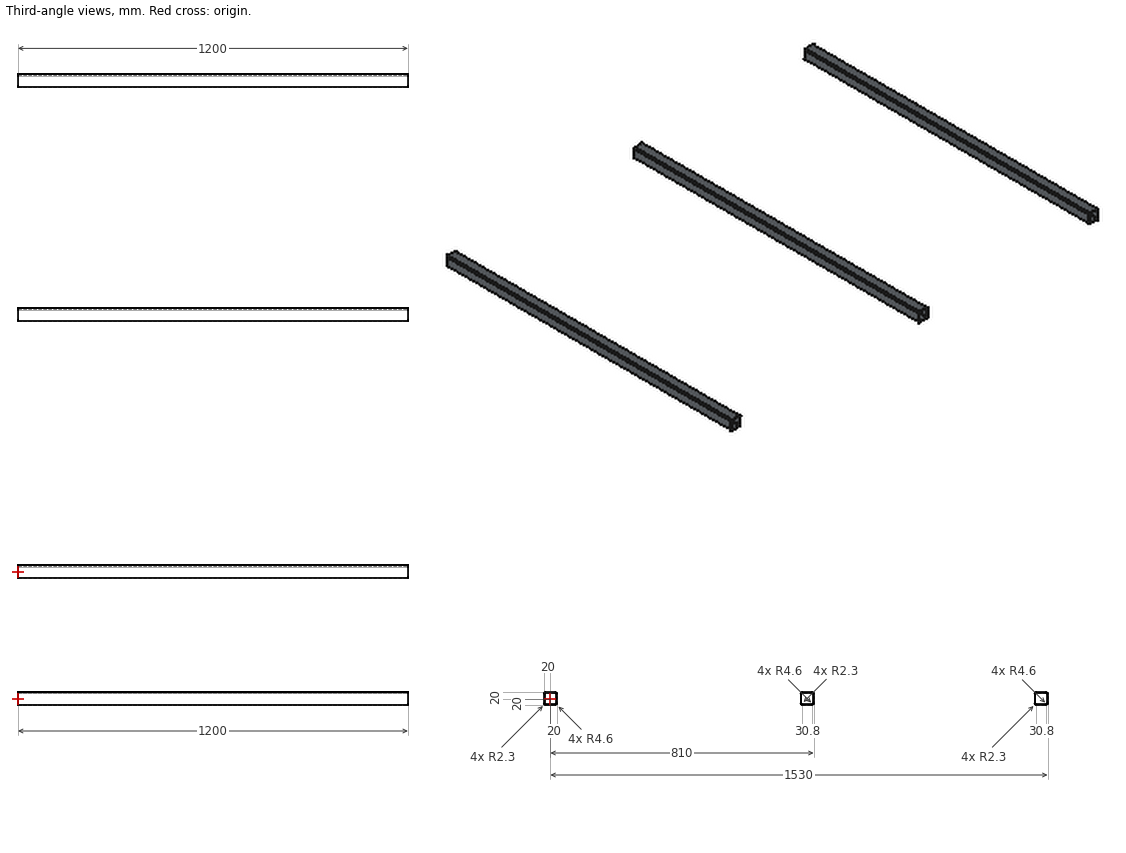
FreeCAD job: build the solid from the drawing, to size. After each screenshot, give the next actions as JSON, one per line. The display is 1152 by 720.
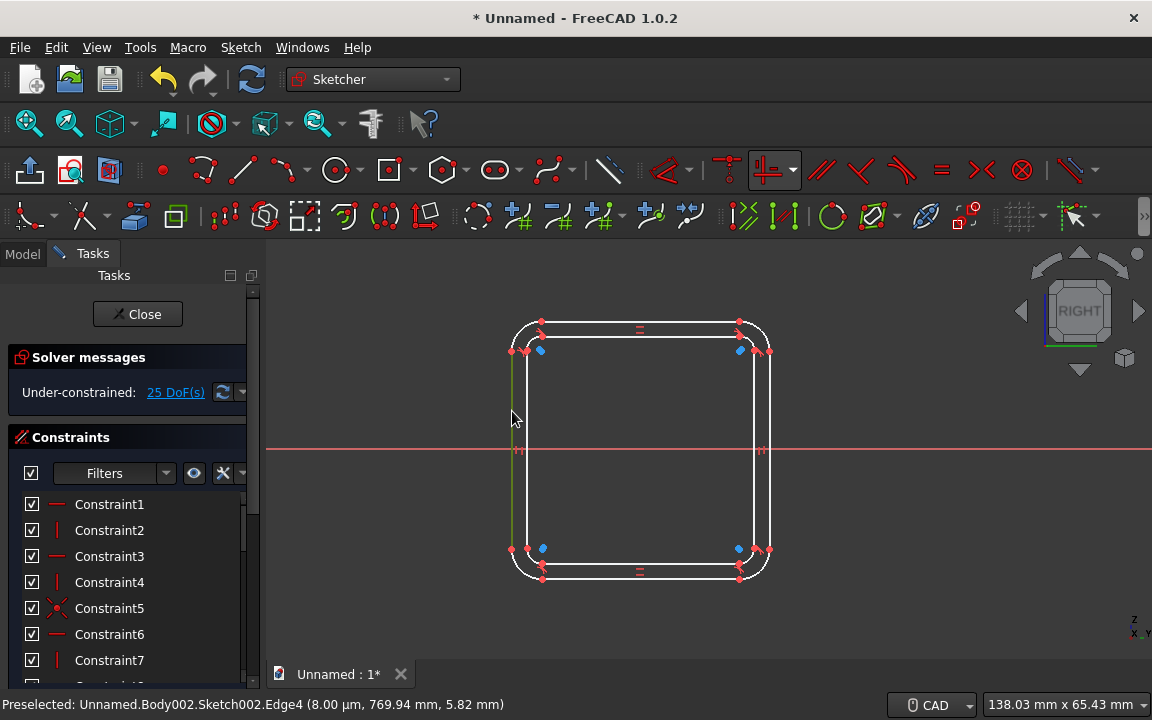
{"action": "left_click", "coordinate": [515, 563]}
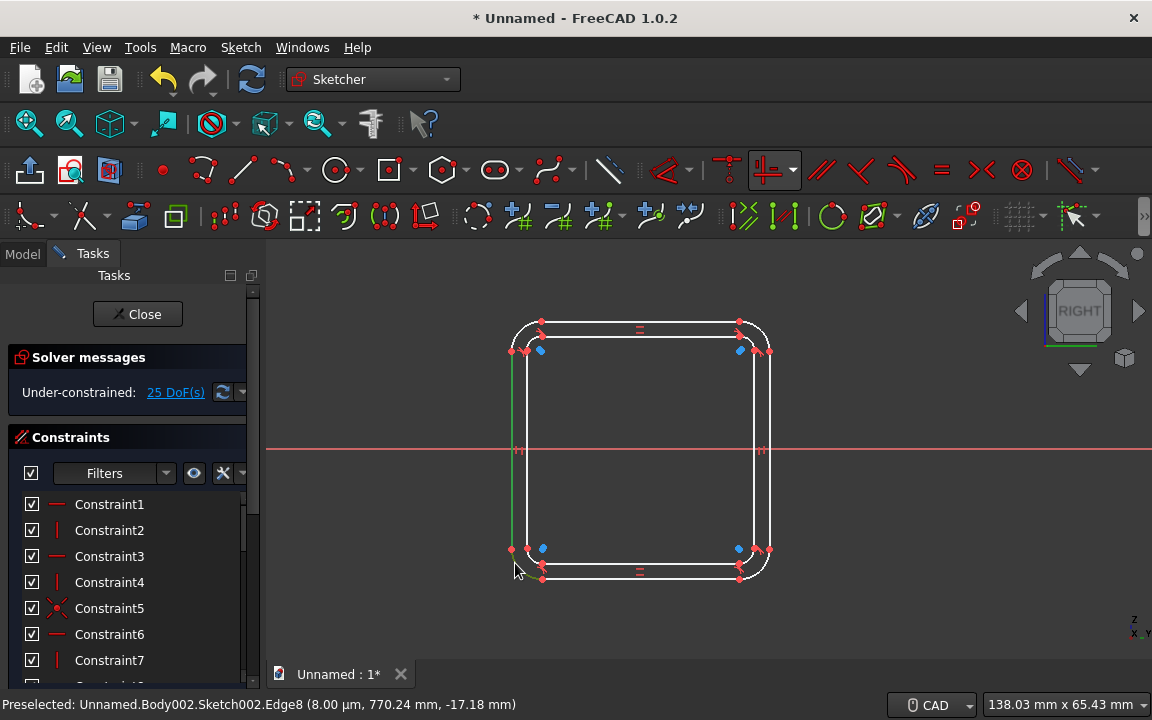
{"action": "key", "text": "t"}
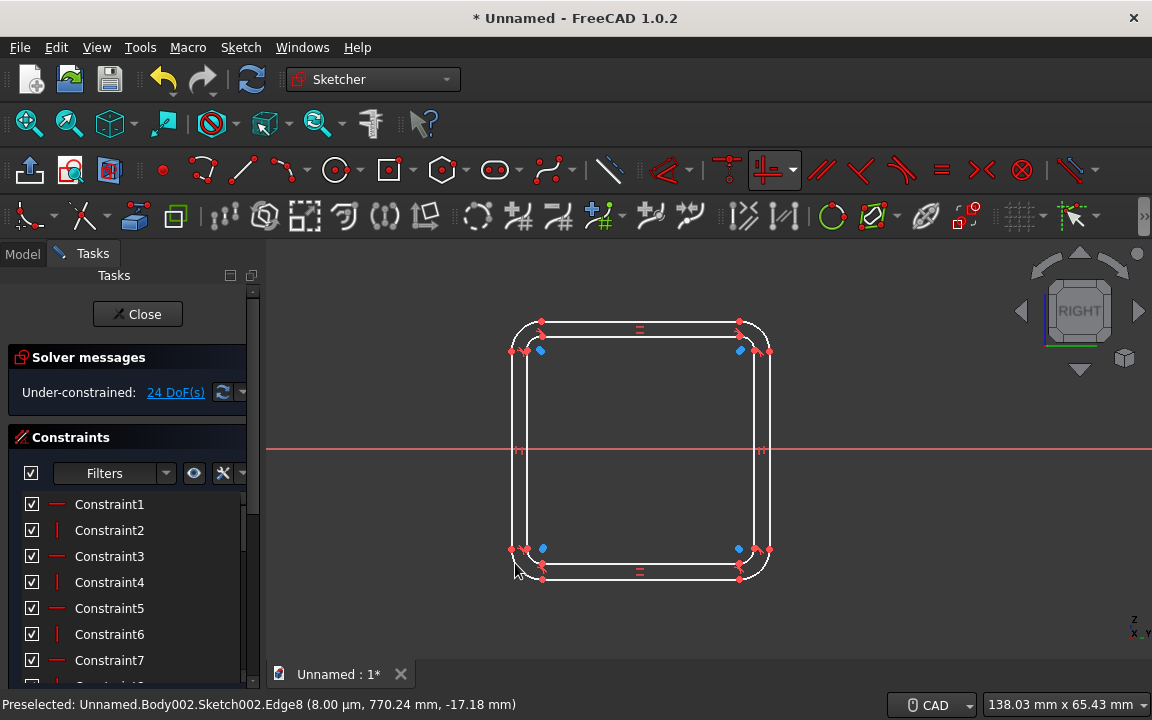
{"action": "left_click", "coordinate": [680, 564]}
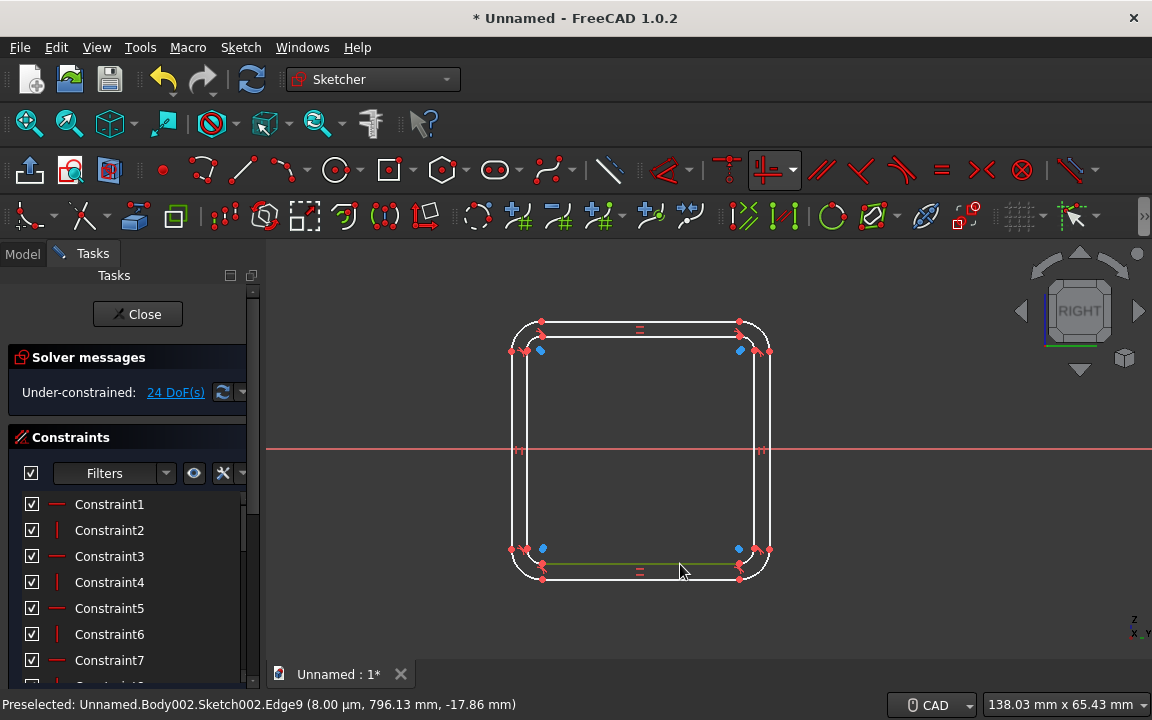
{"action": "left_click", "coordinate": [532, 559]}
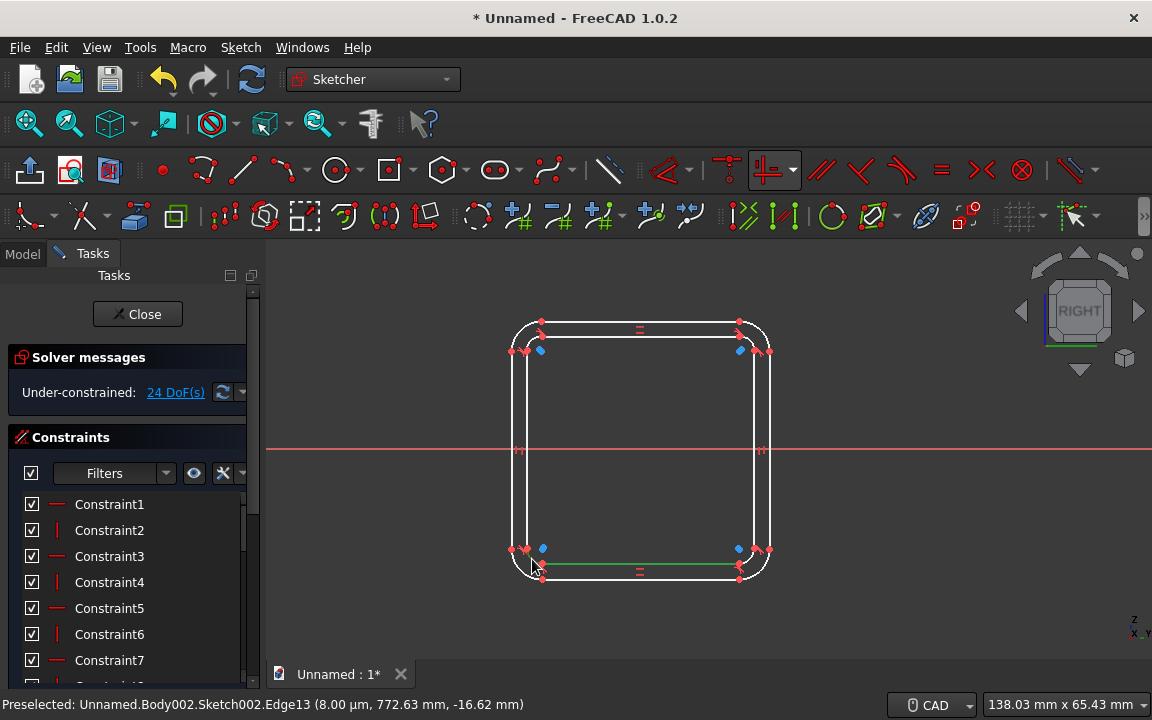
{"action": "key", "text": "t"}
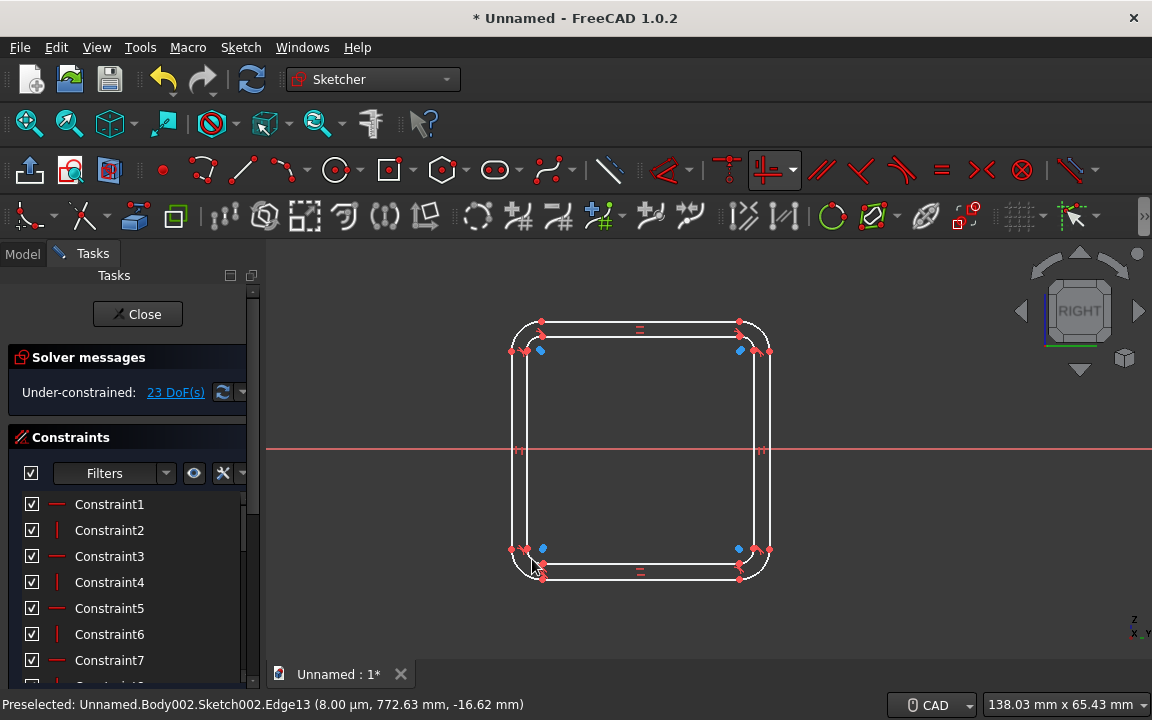
{"action": "left_click", "coordinate": [680, 564]}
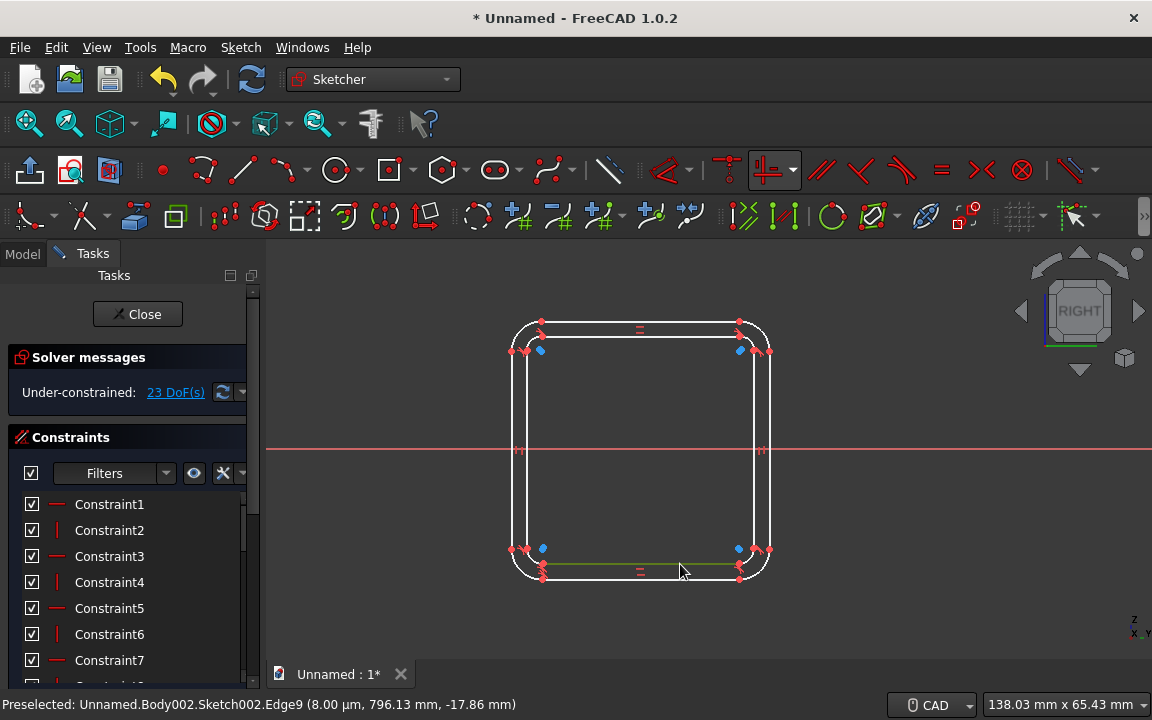
{"action": "left_click", "coordinate": [749, 559]}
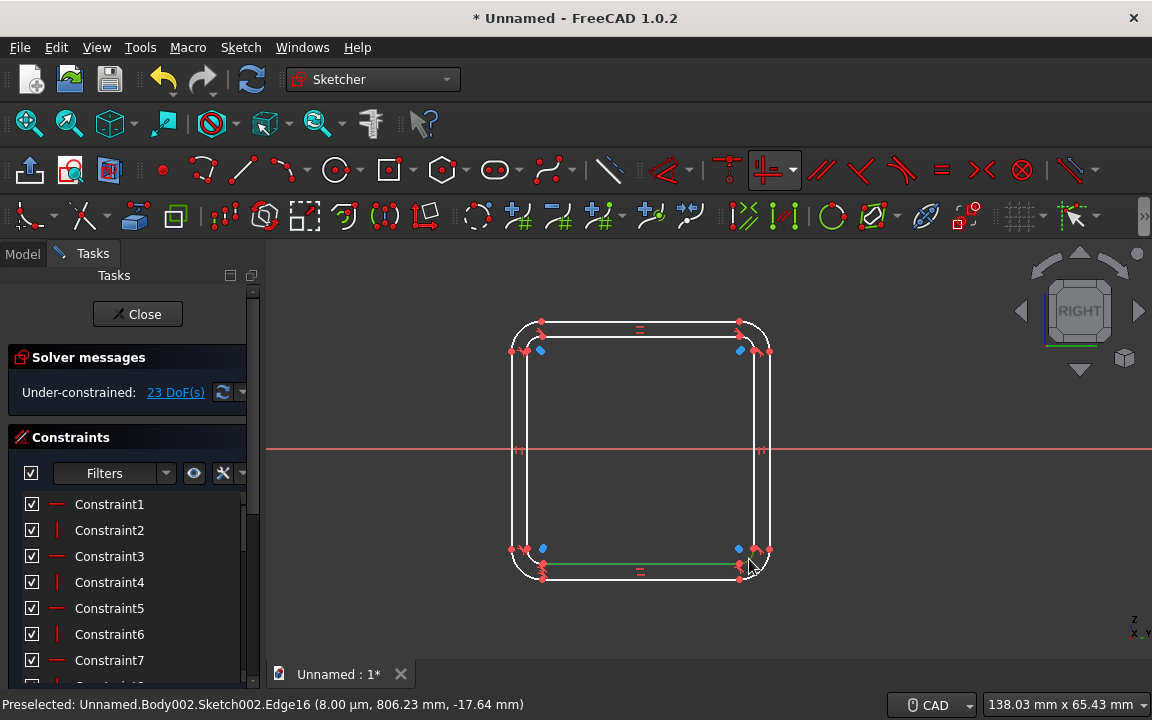
{"action": "key", "text": "t"}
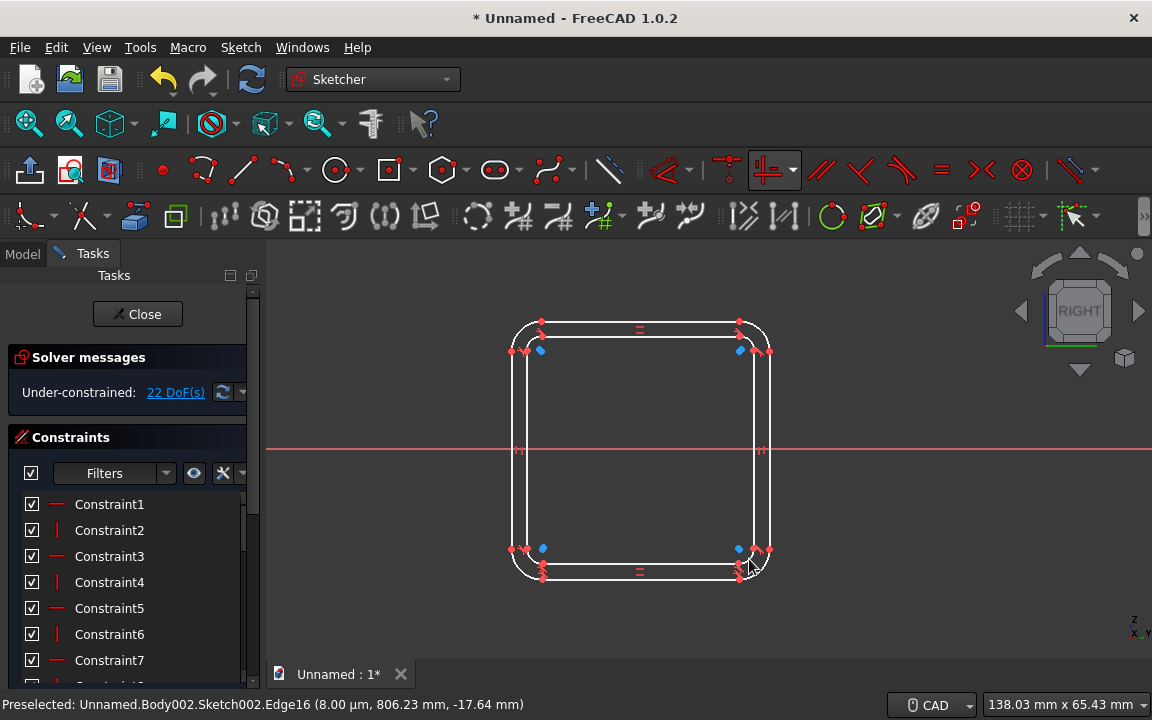
{"action": "left_click", "coordinate": [527, 490]}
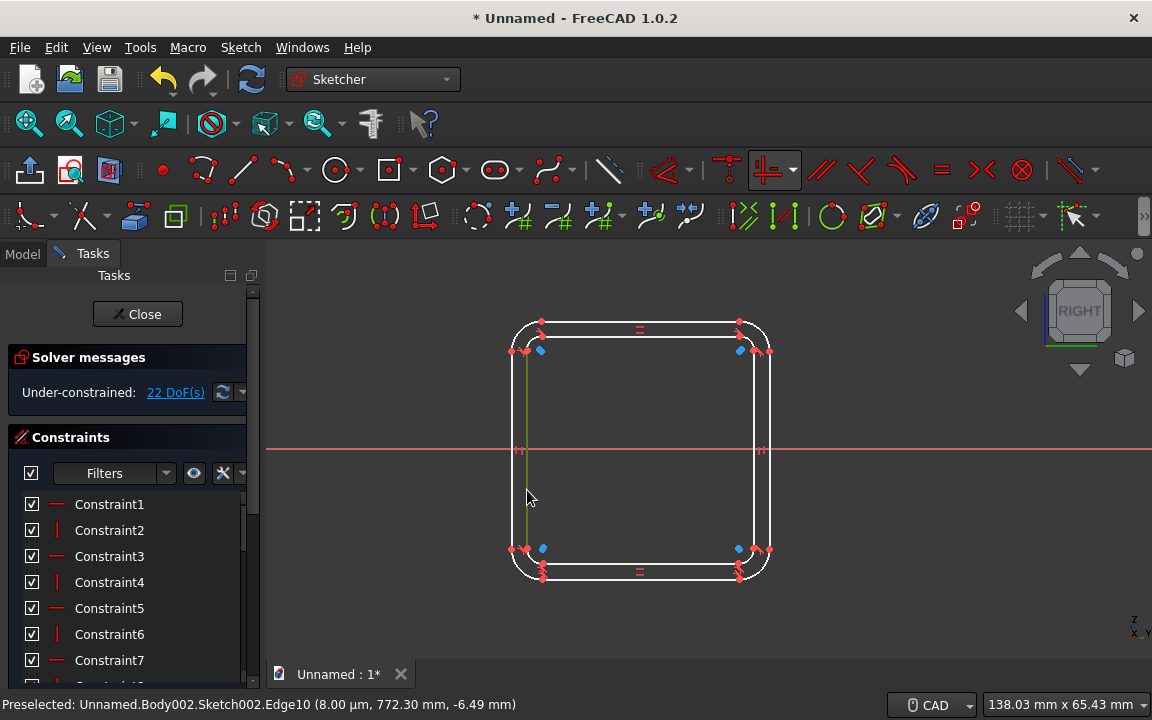
{"action": "left_click", "coordinate": [532, 560]}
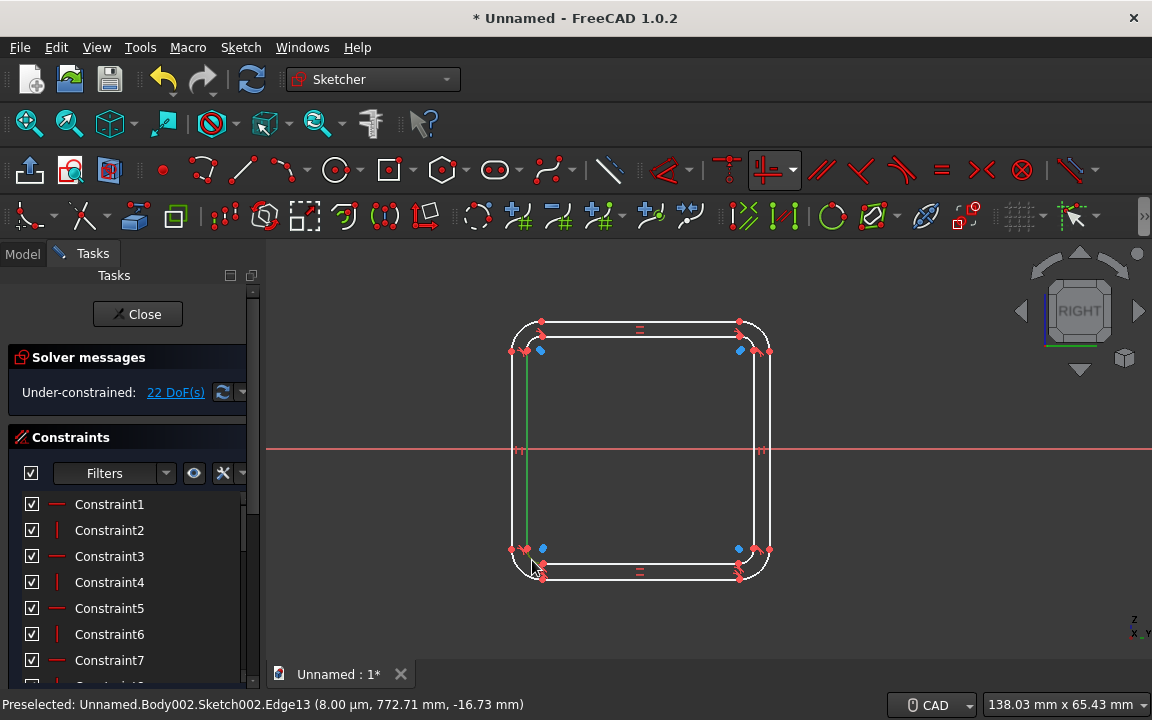
{"action": "key", "text": "t"}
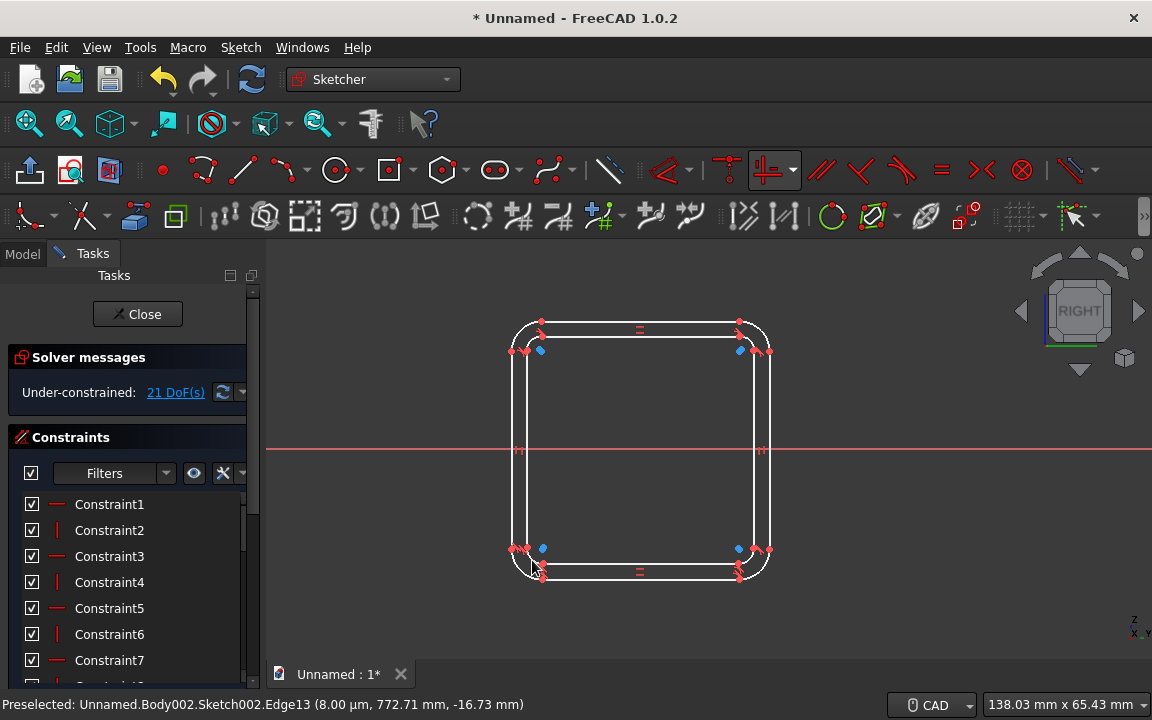
{"action": "left_click", "coordinate": [527, 489]}